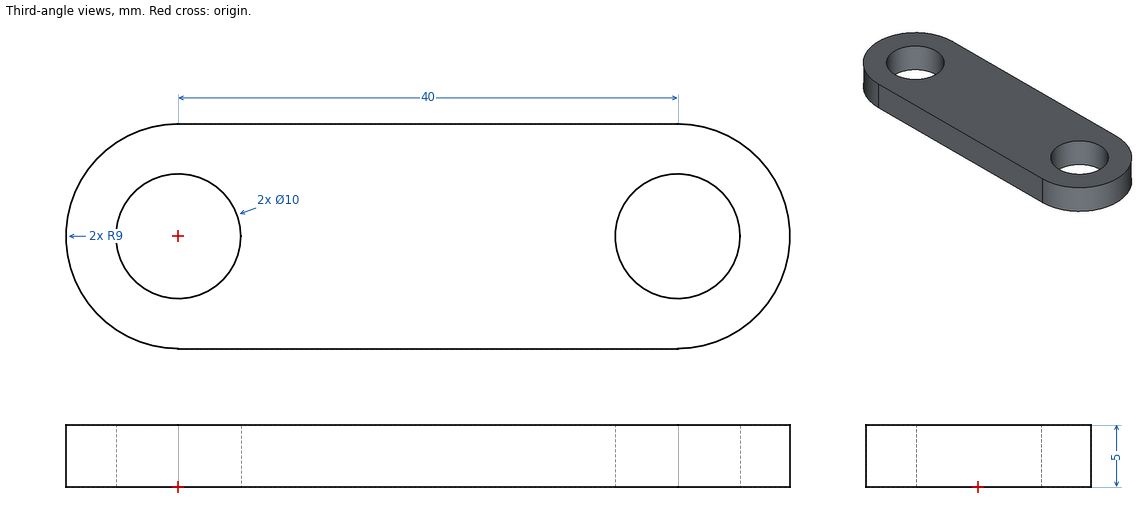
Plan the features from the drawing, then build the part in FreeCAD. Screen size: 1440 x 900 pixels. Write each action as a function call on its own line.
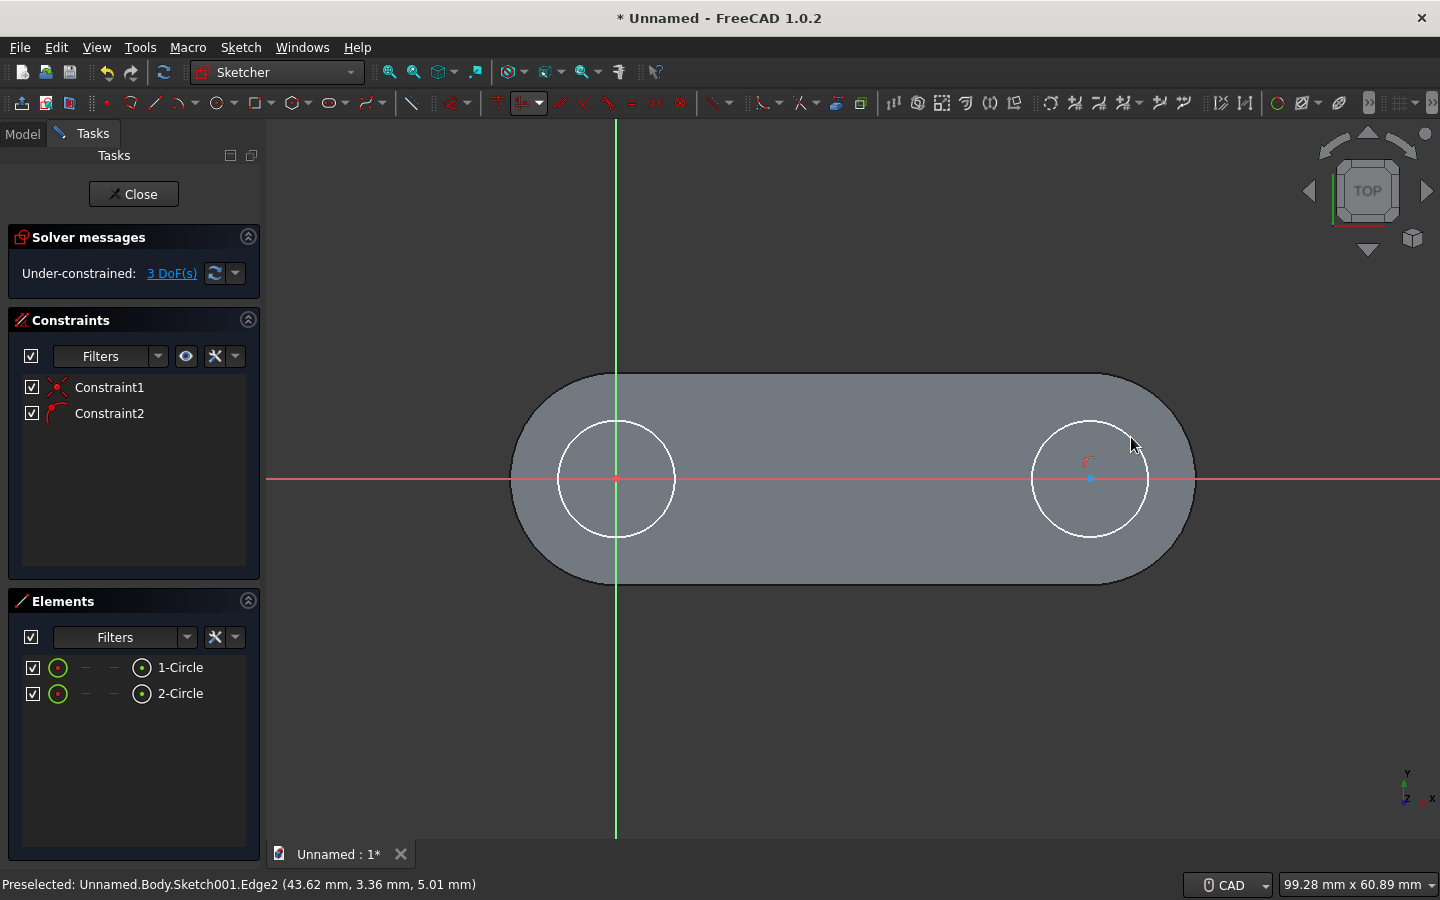
click(658, 438)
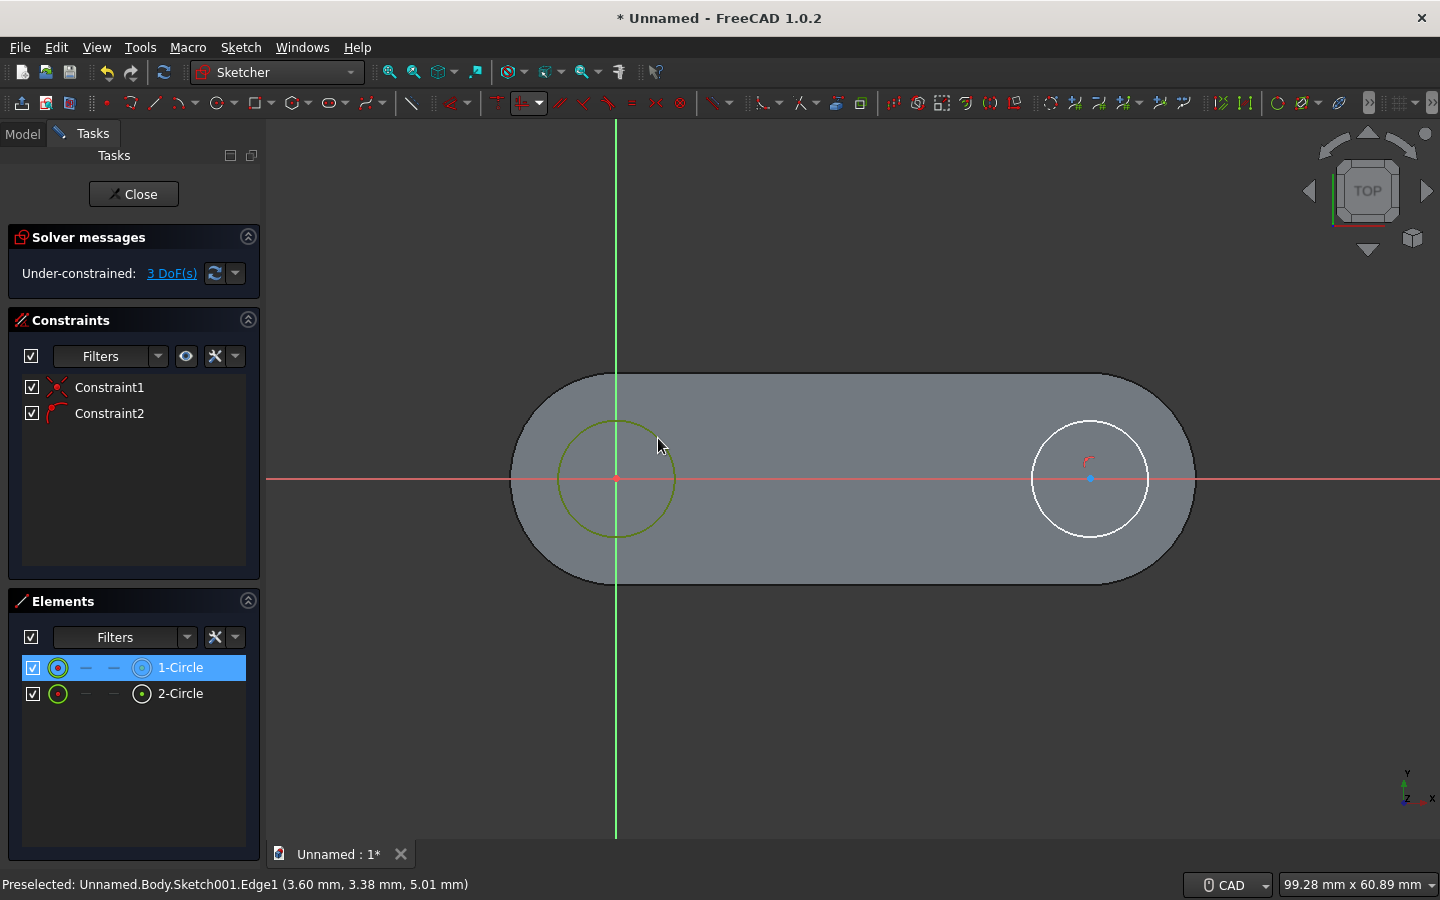
click(1131, 438)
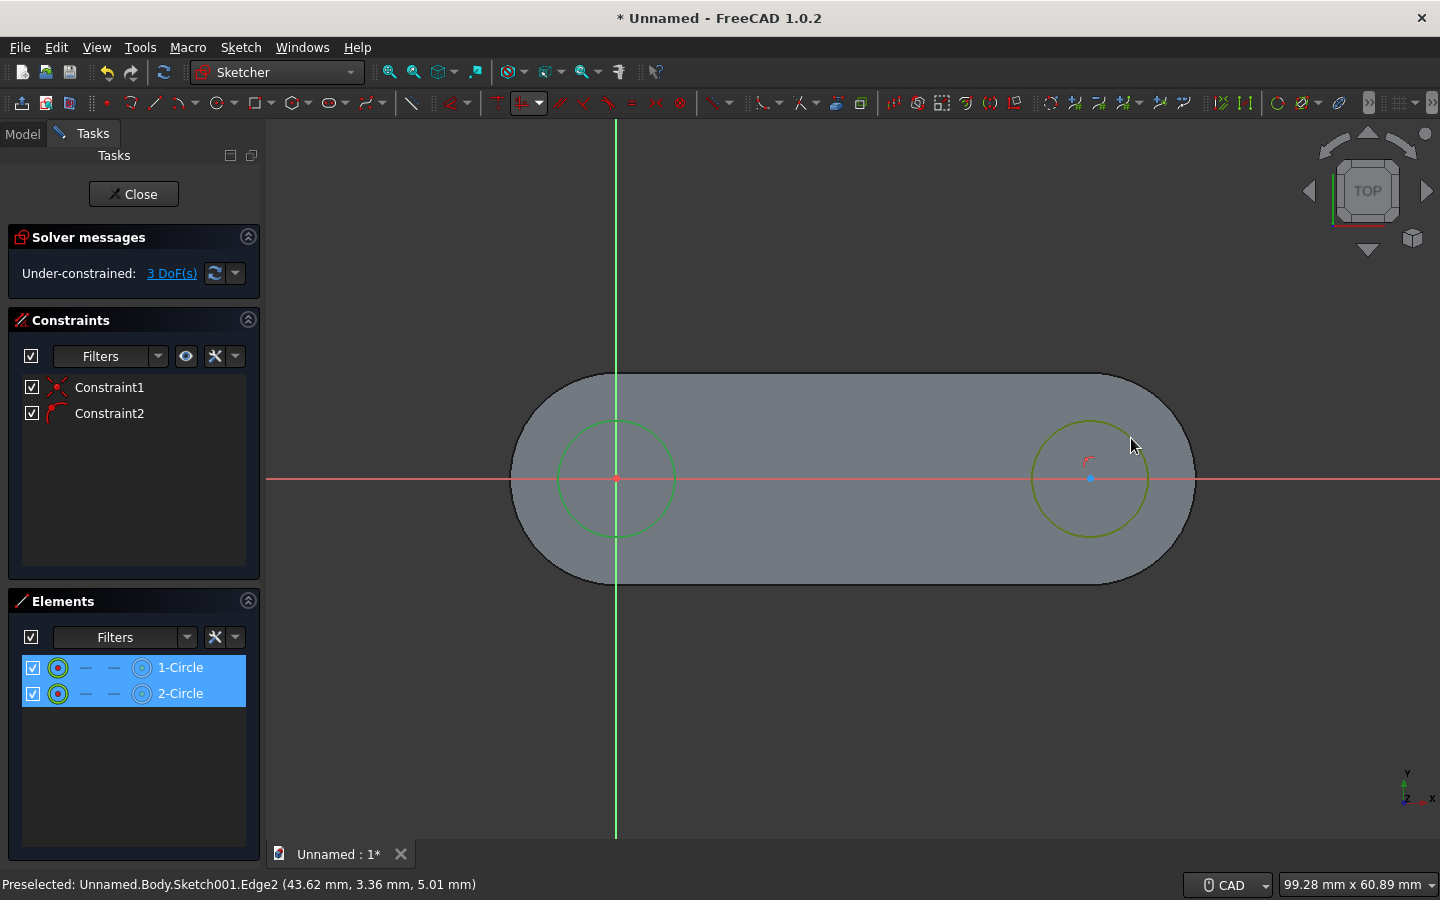
click(632, 104)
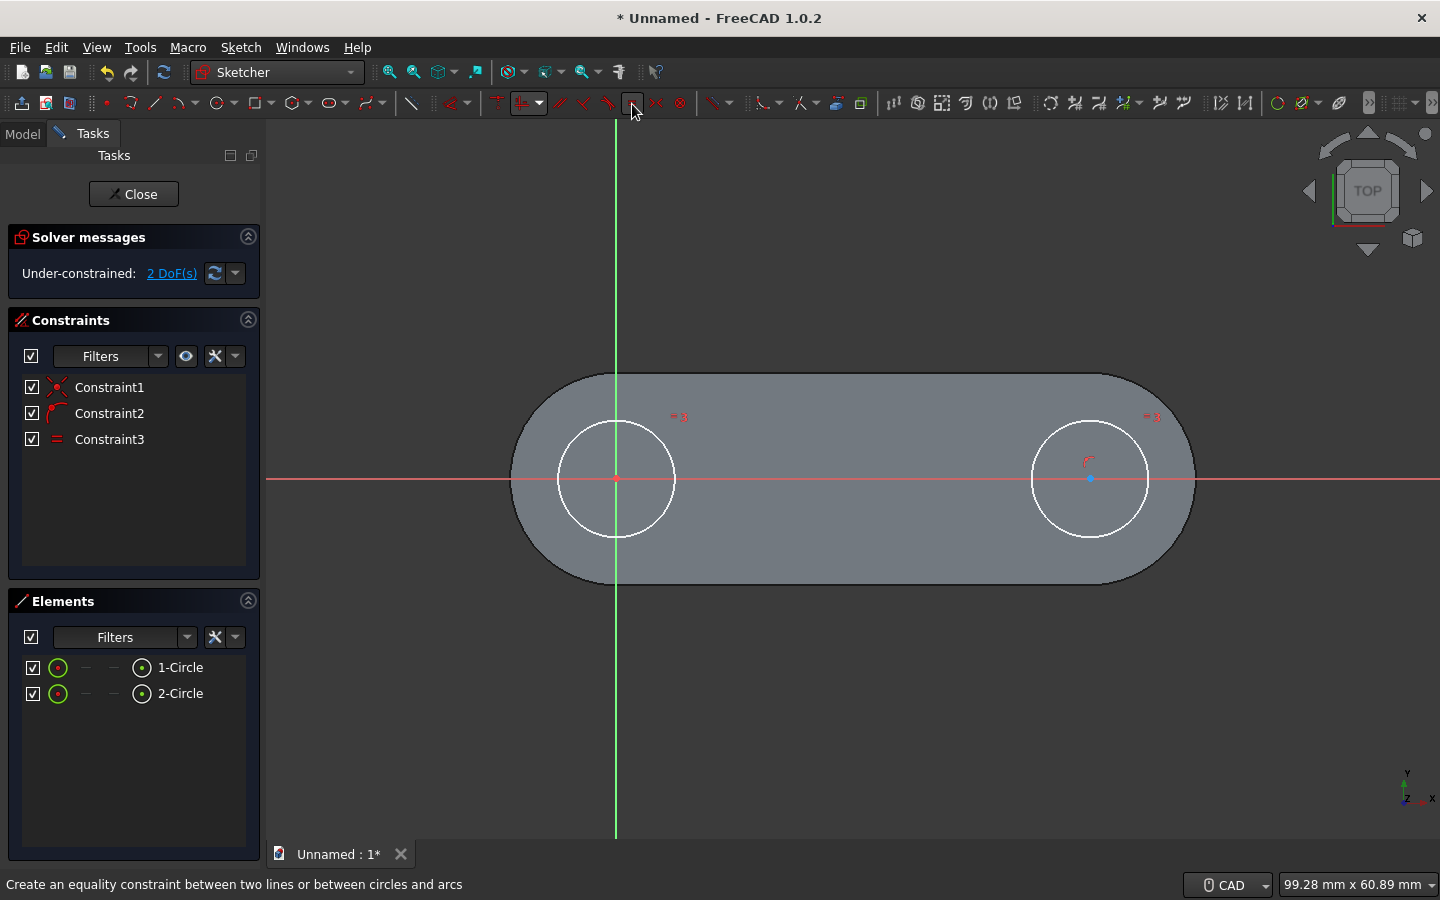
key(d)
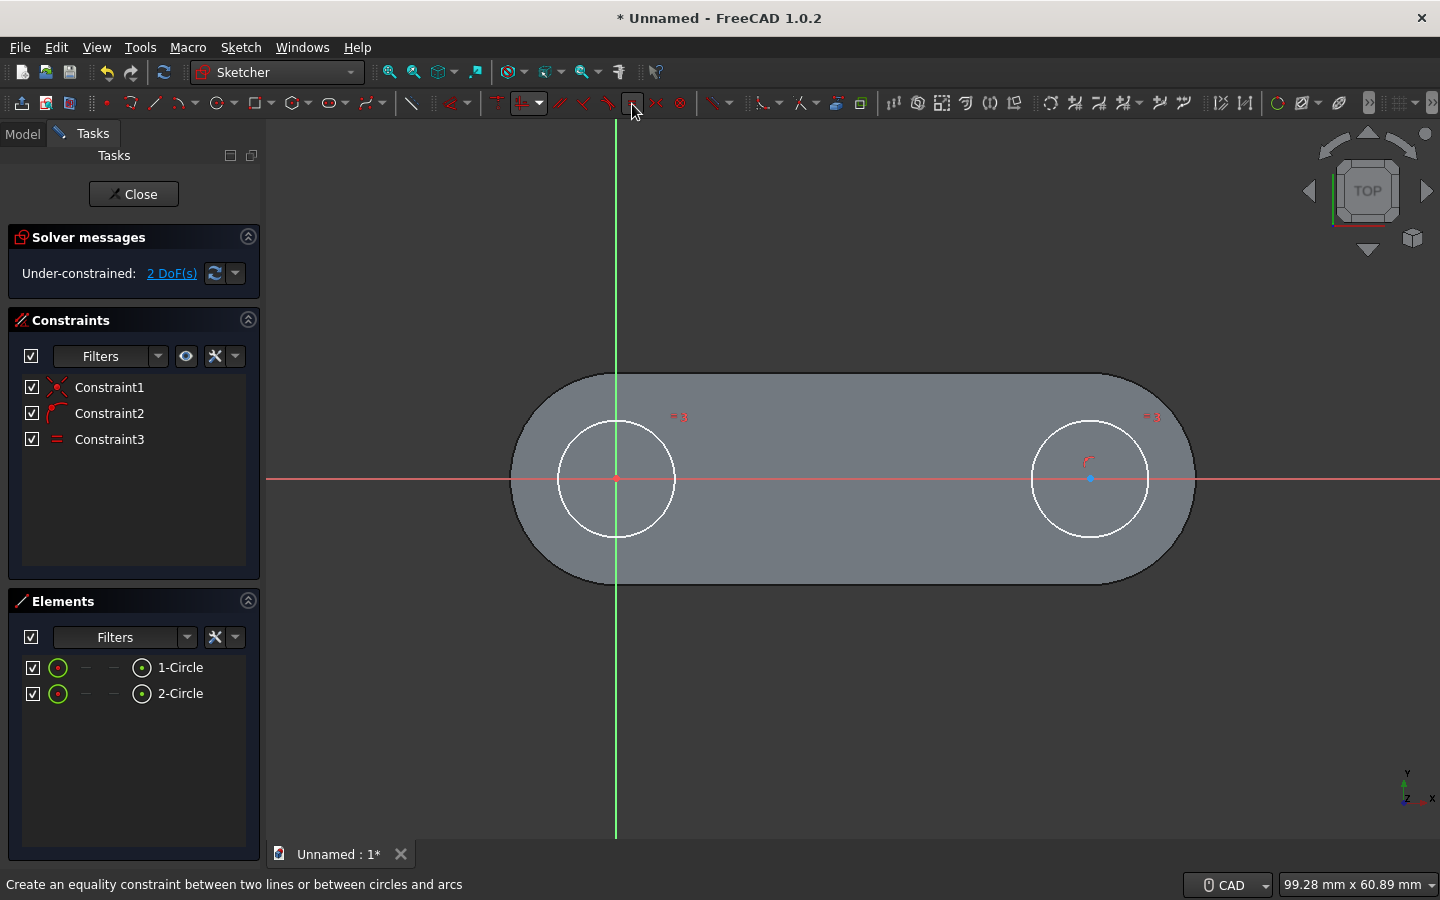
click(658, 438)
click(681, 416)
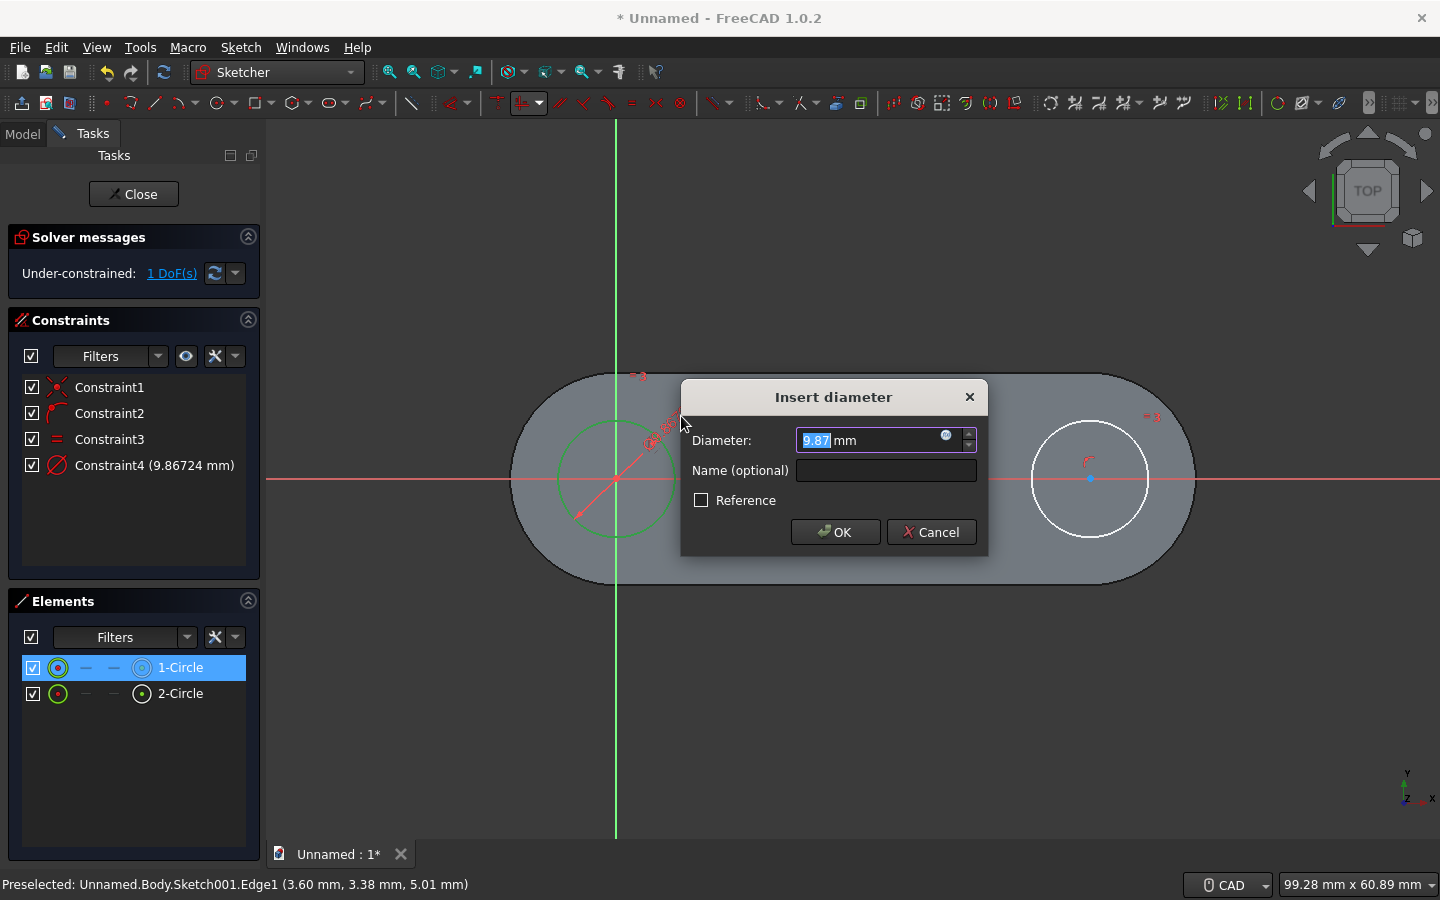
text(10)
key(Return)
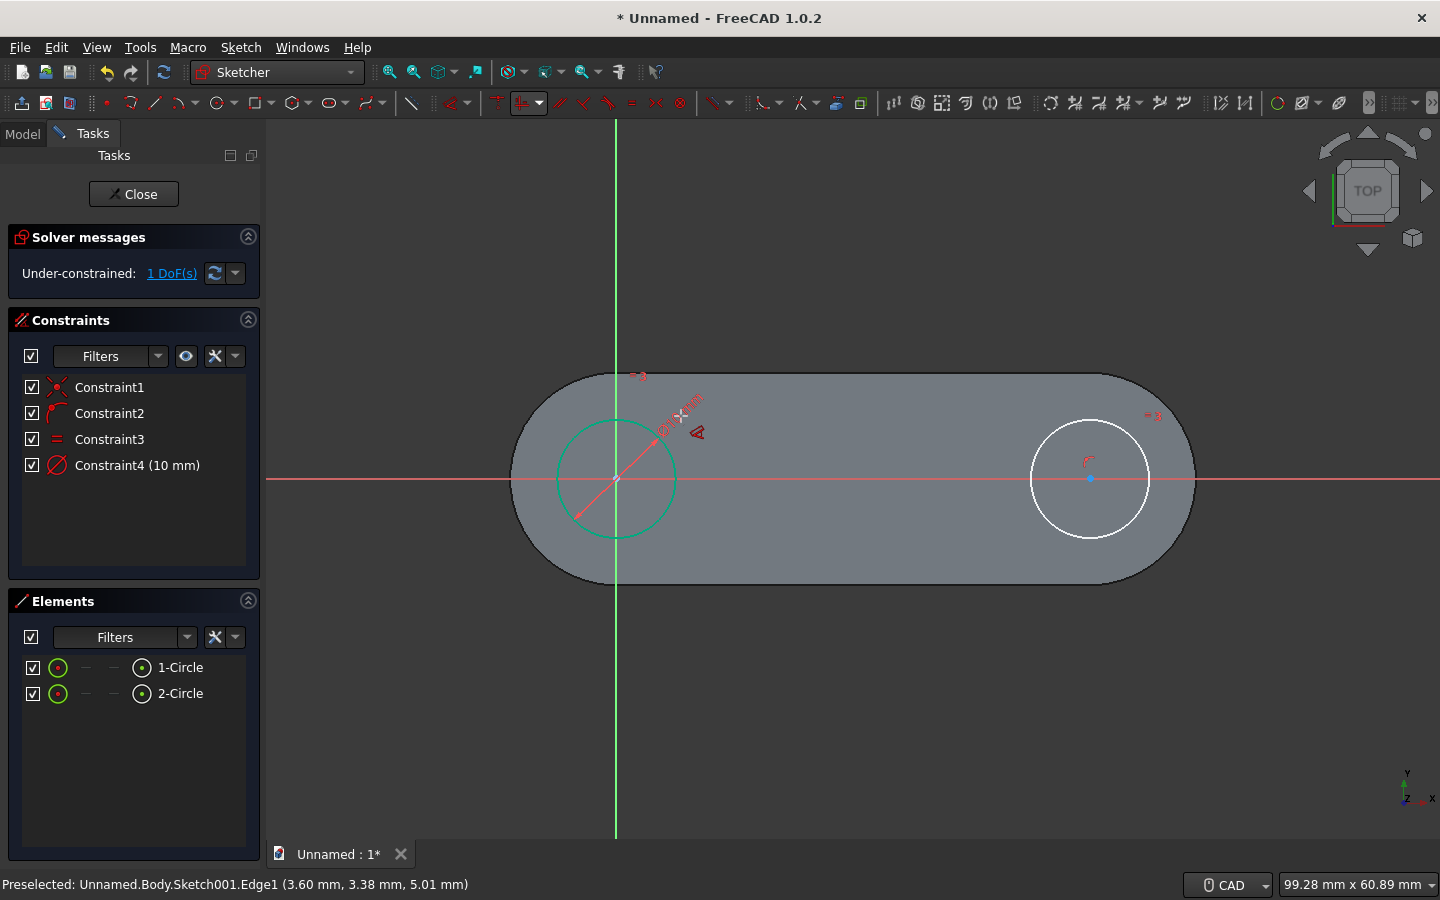
click(1090, 479)
click(853, 513)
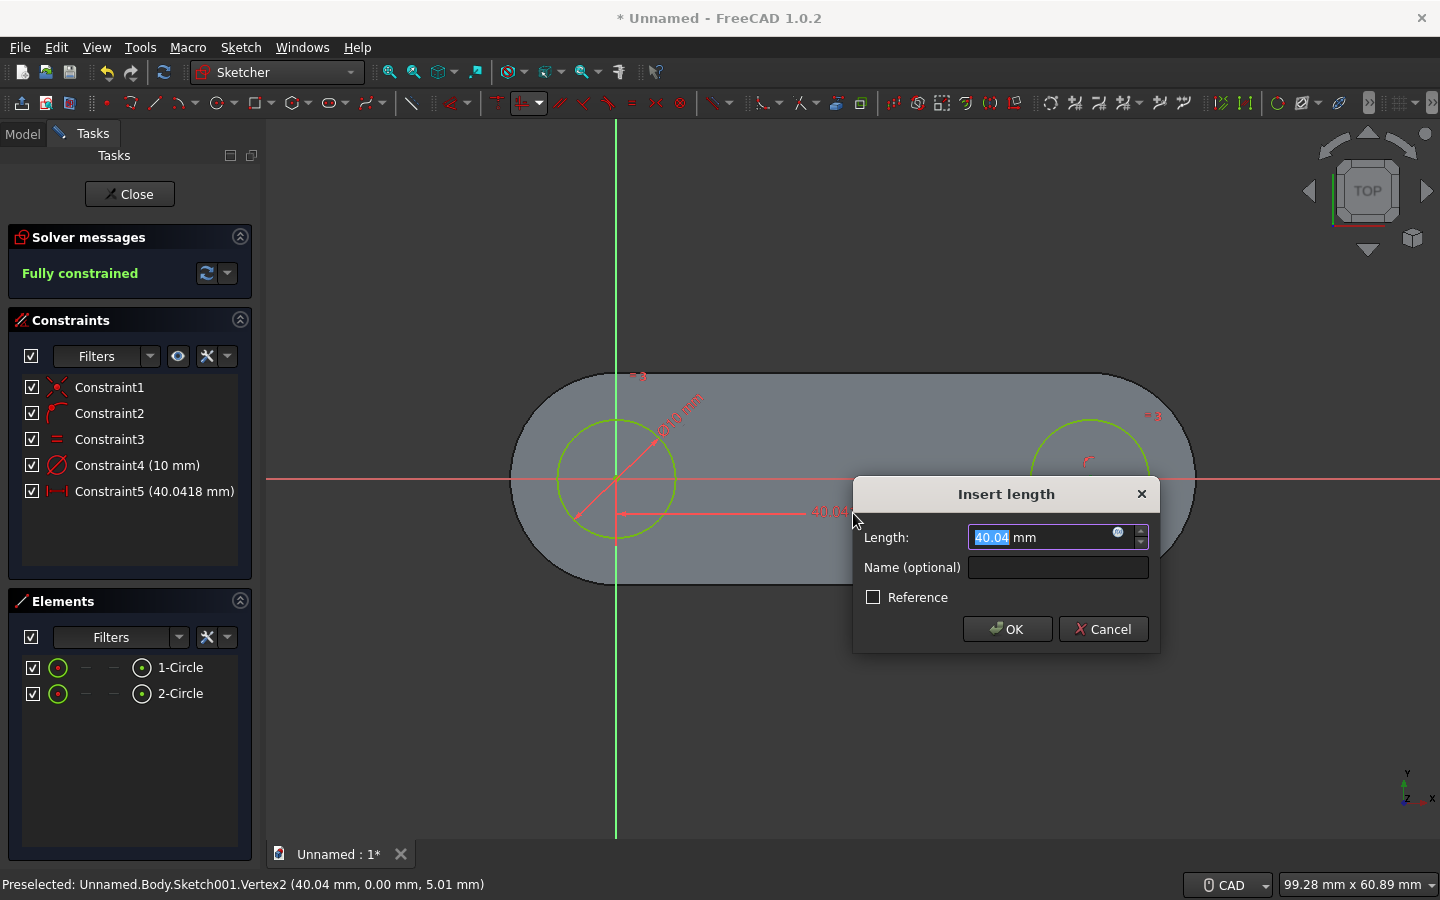
text(40)
key(Return)
key(Escape)